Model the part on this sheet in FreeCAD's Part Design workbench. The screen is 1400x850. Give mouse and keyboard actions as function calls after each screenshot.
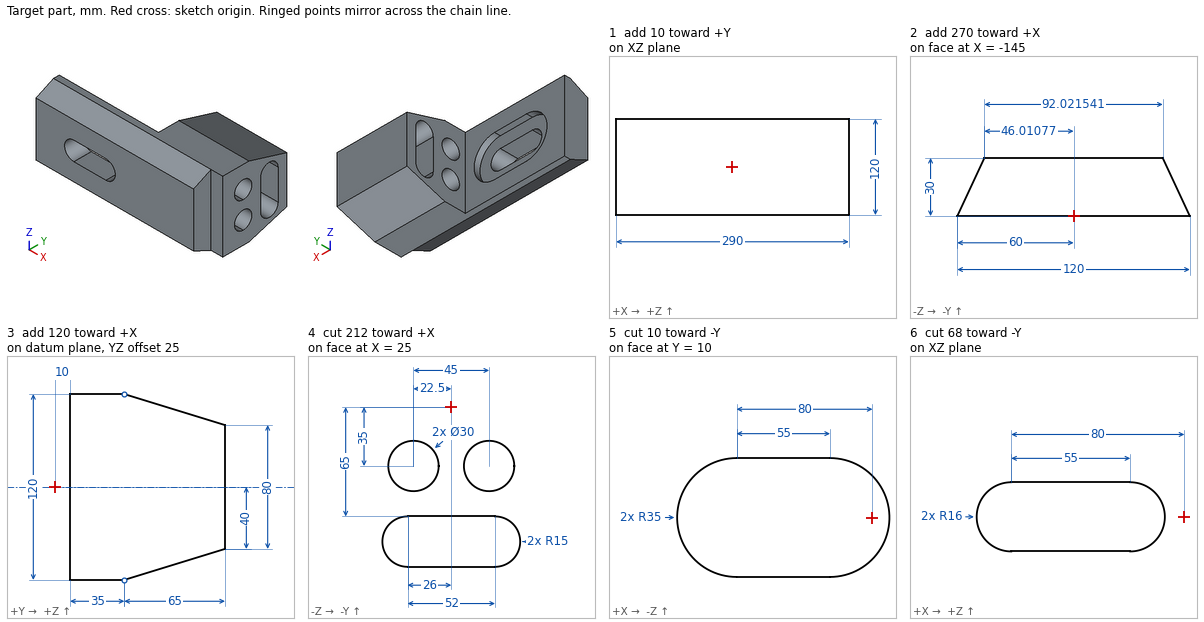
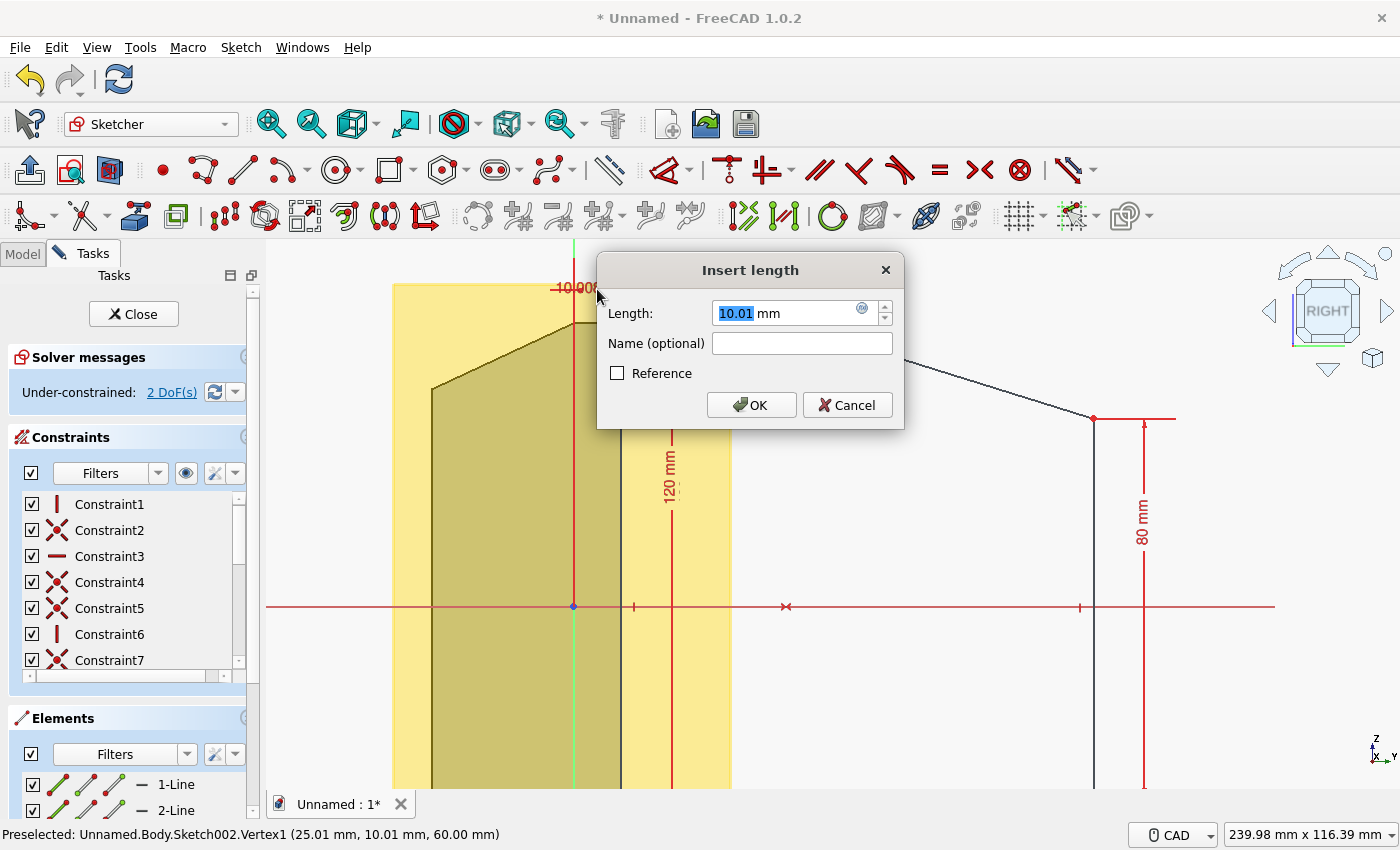
text(10)
key(Return)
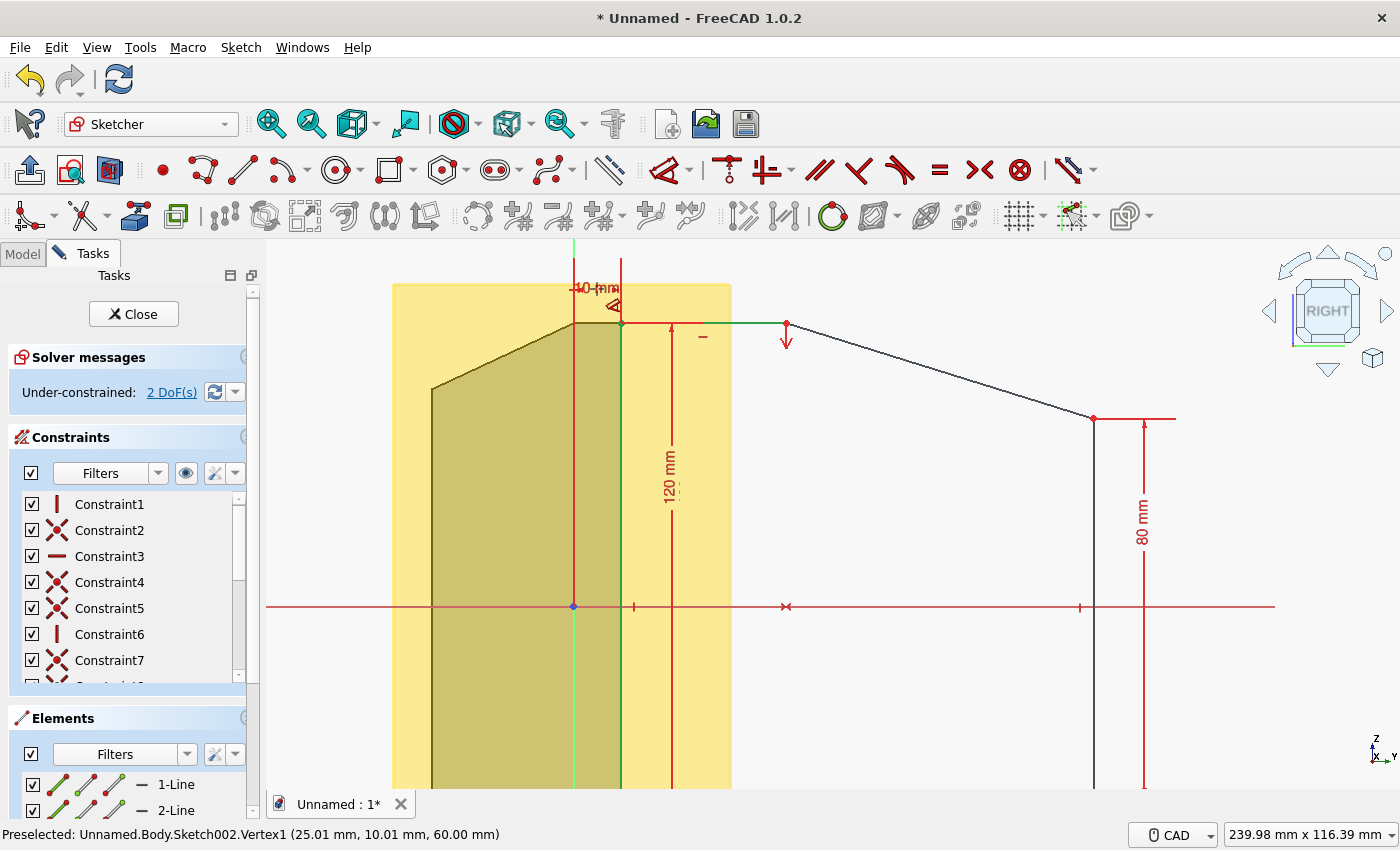
scroll(624, 325, down, 2)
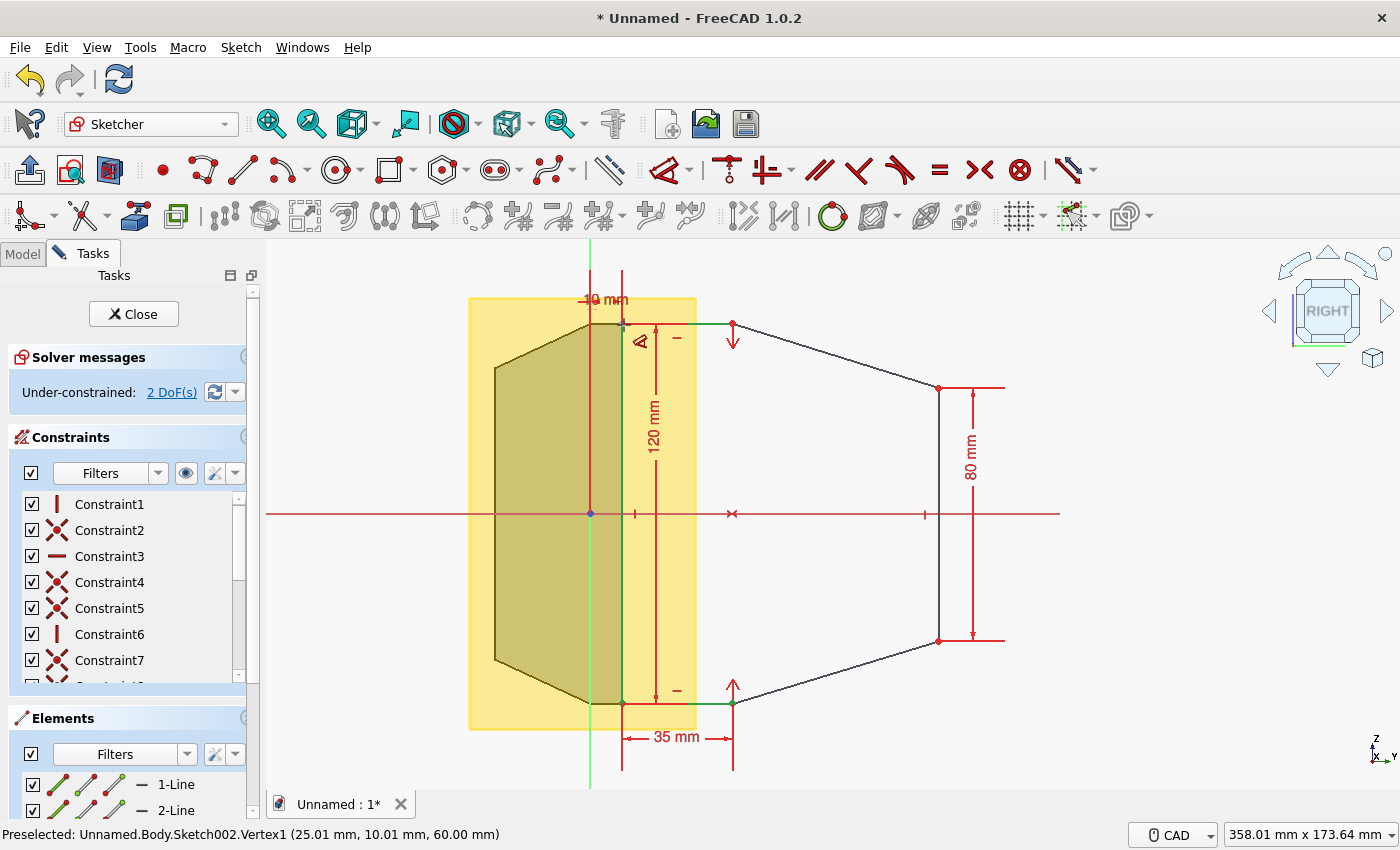
click(939, 641)
click(973, 578)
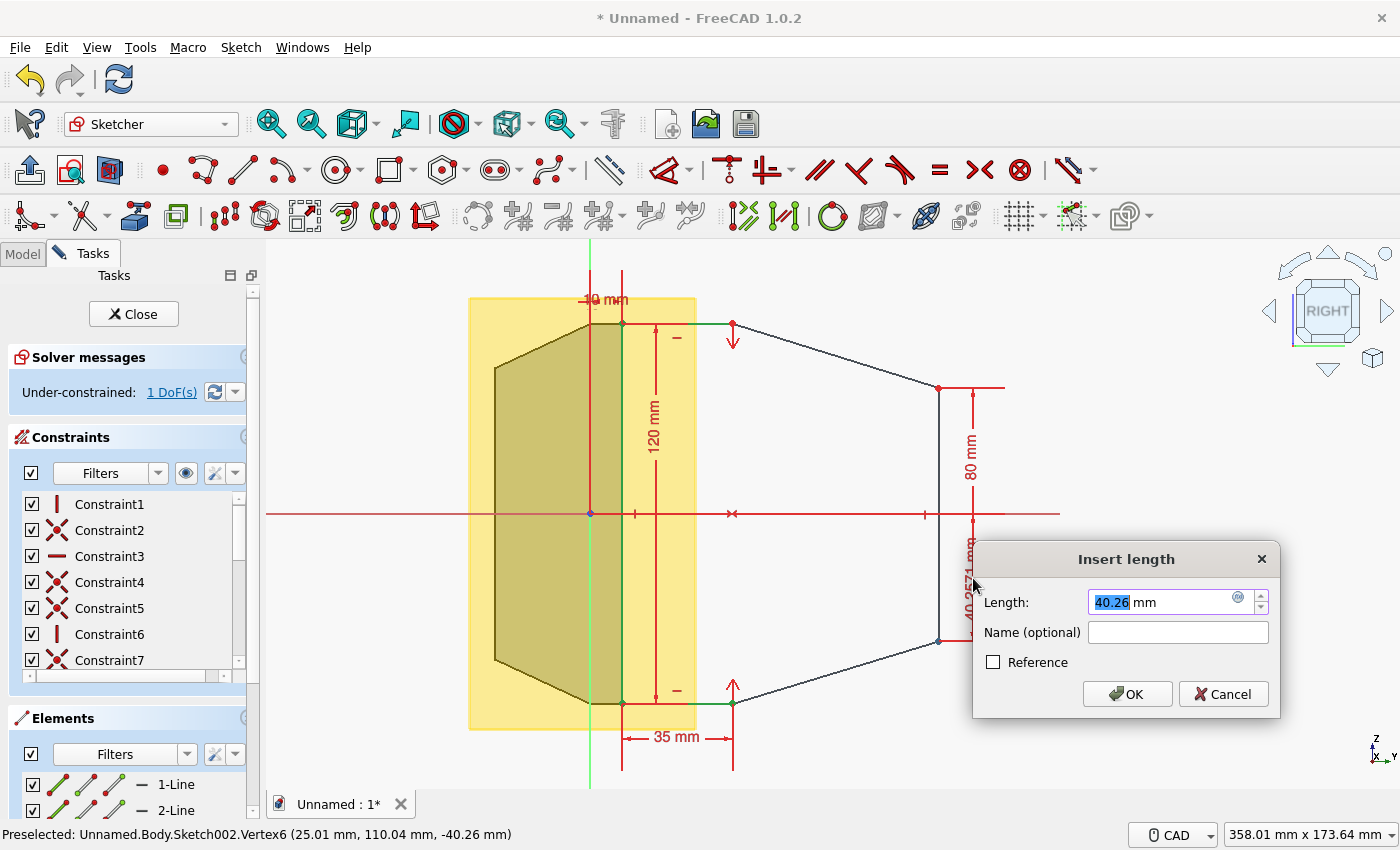
text(40)
key(Return)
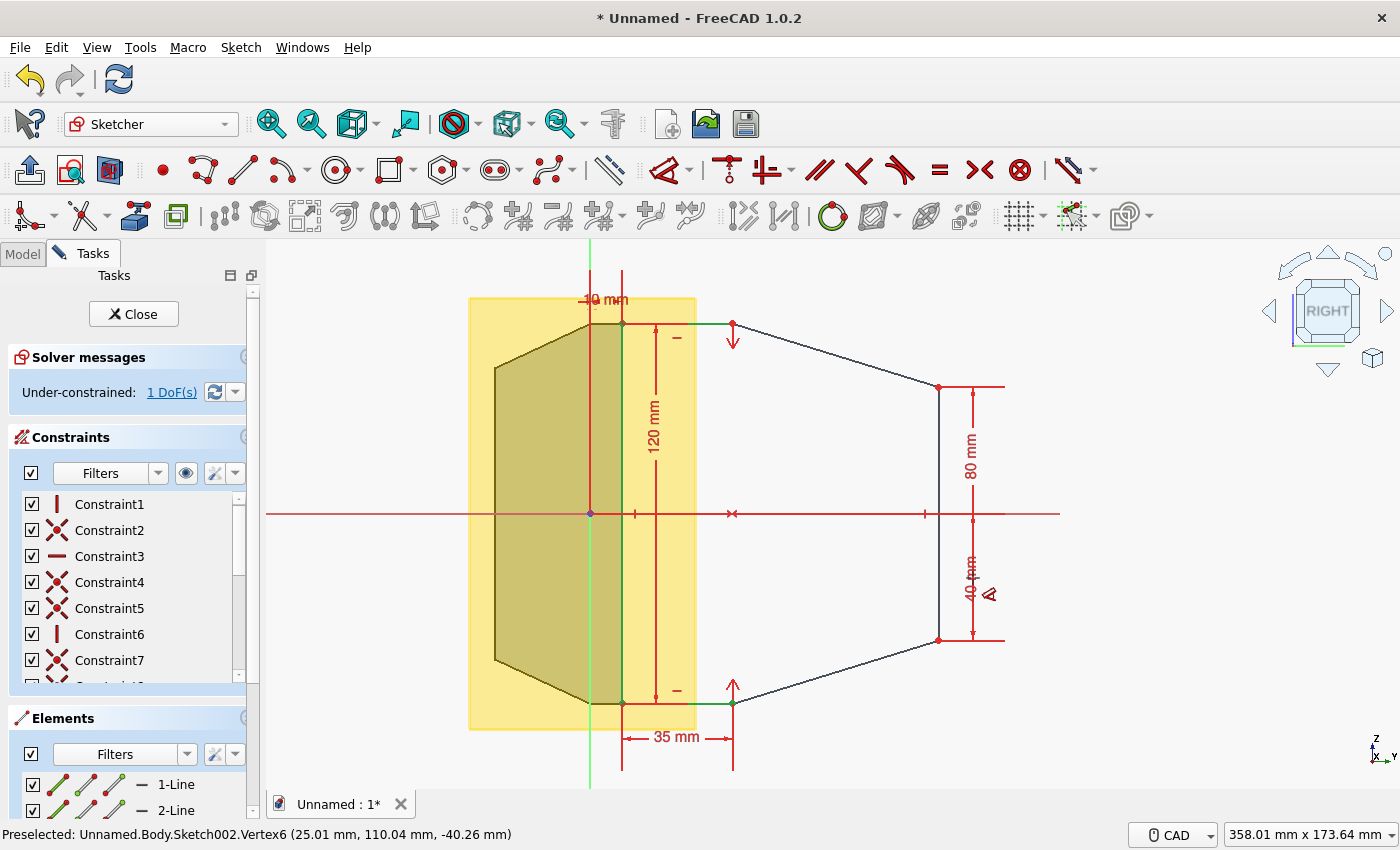
click(795, 685)
click(836, 738)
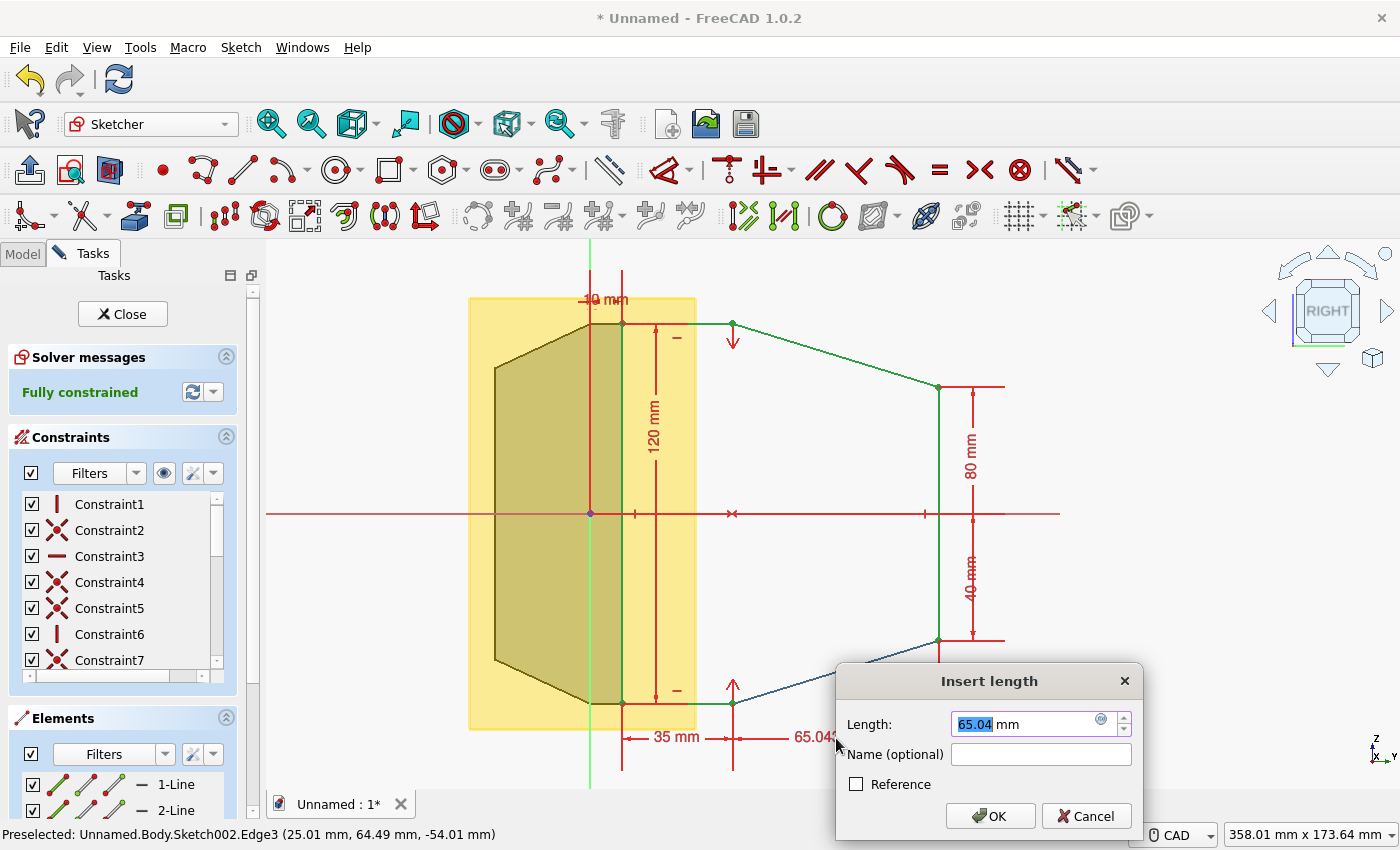
text(65)
key(Return)
key(Escape)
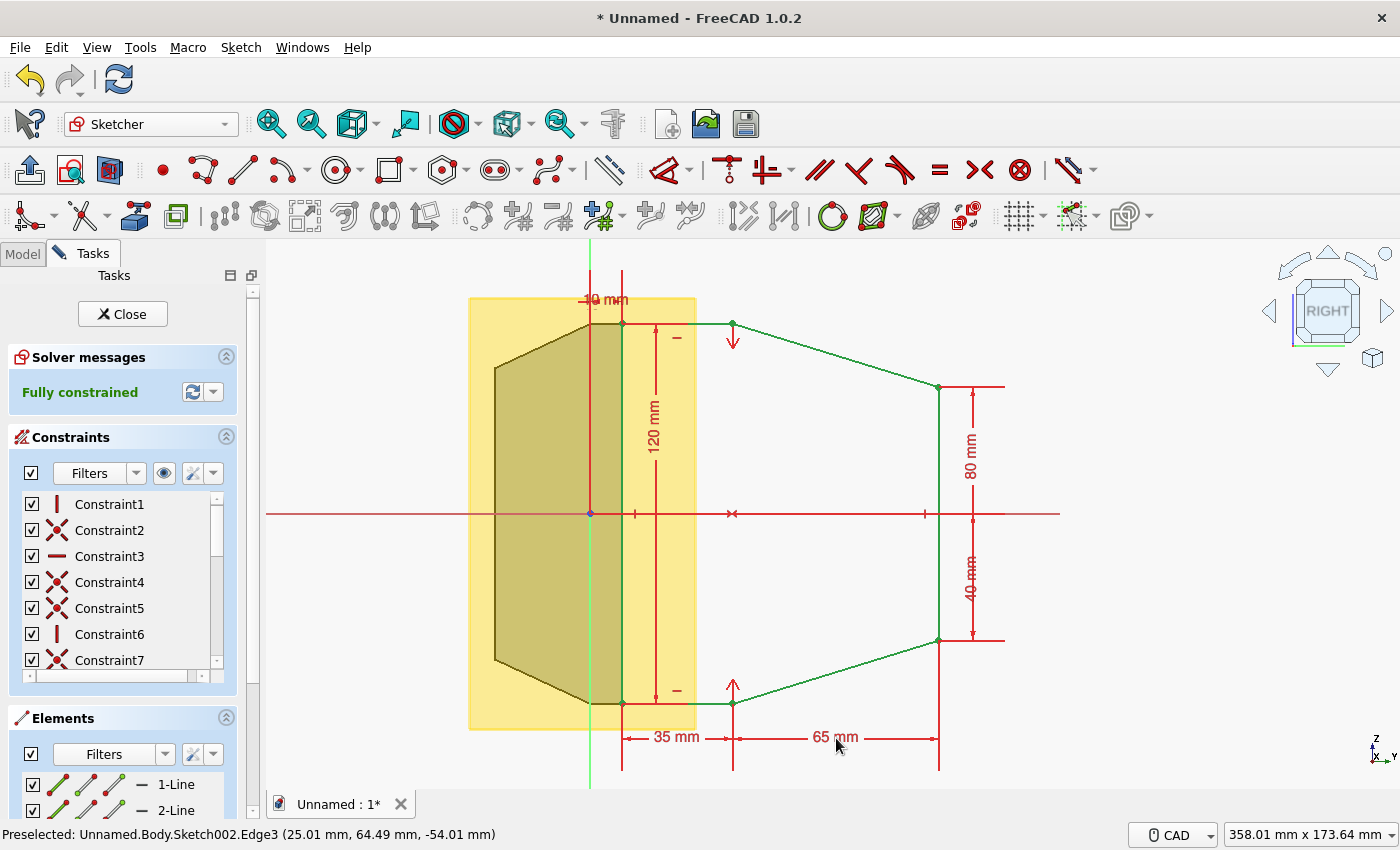
click(123, 314)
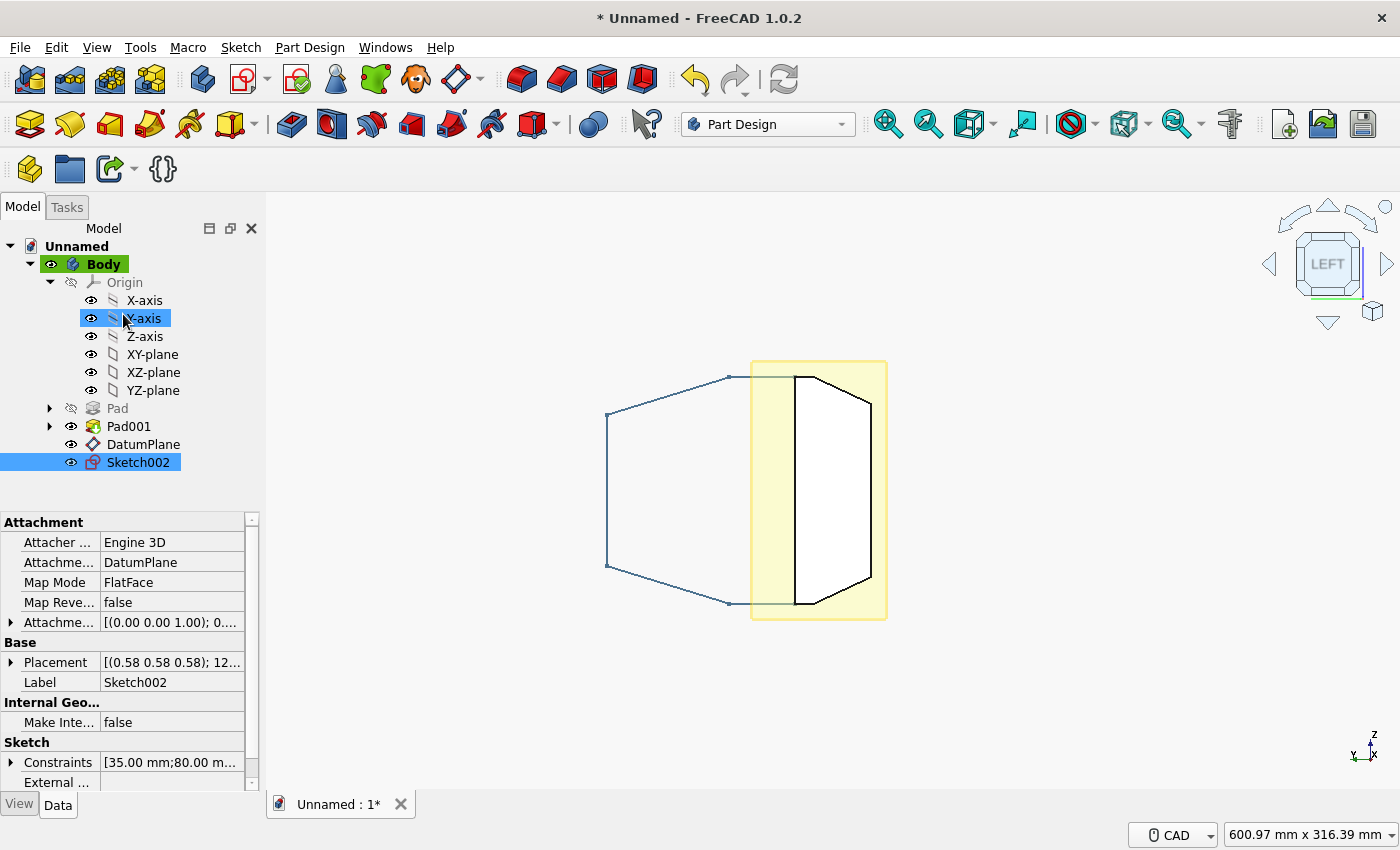
click(30, 124)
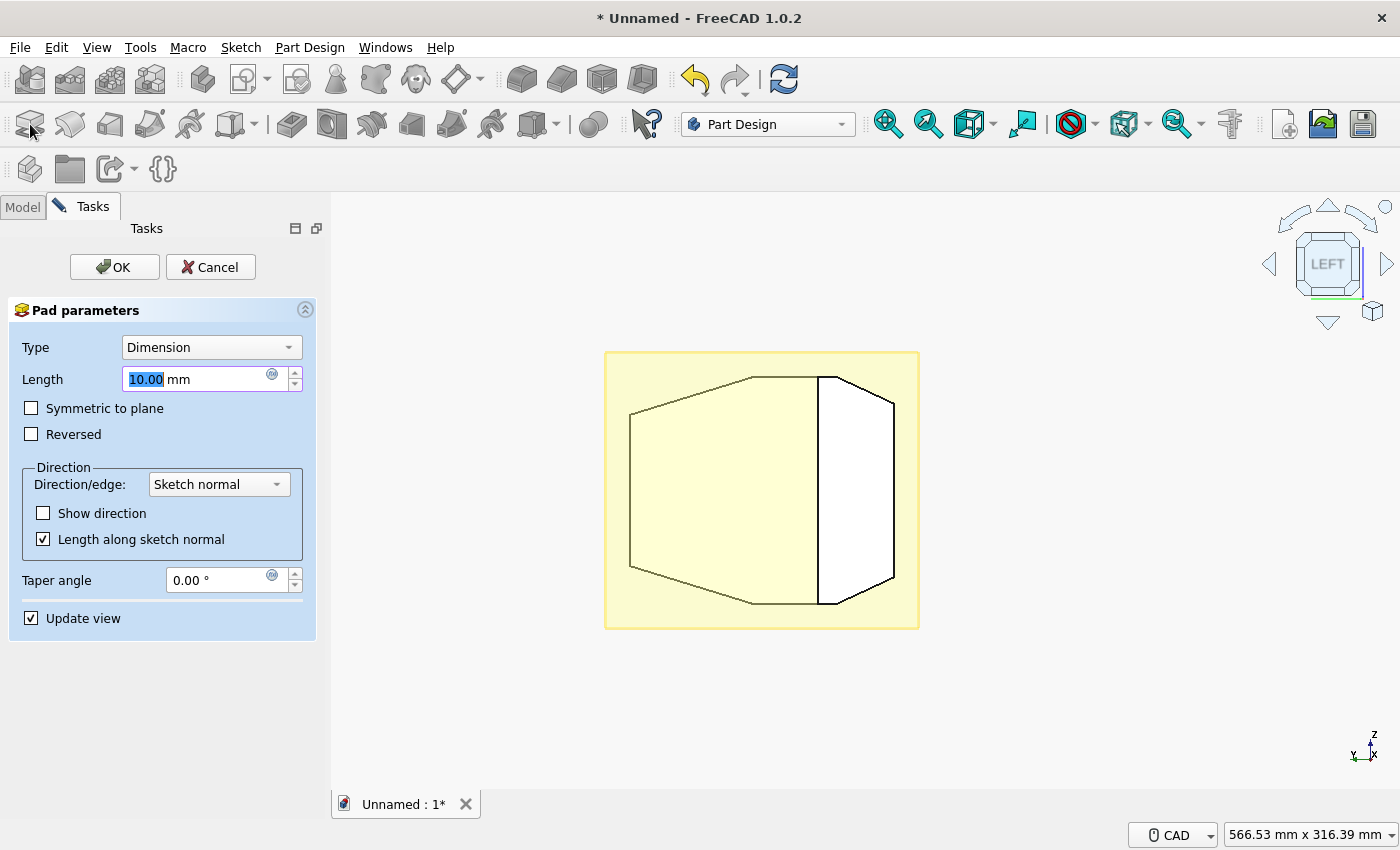
text(120)
key(Tab)